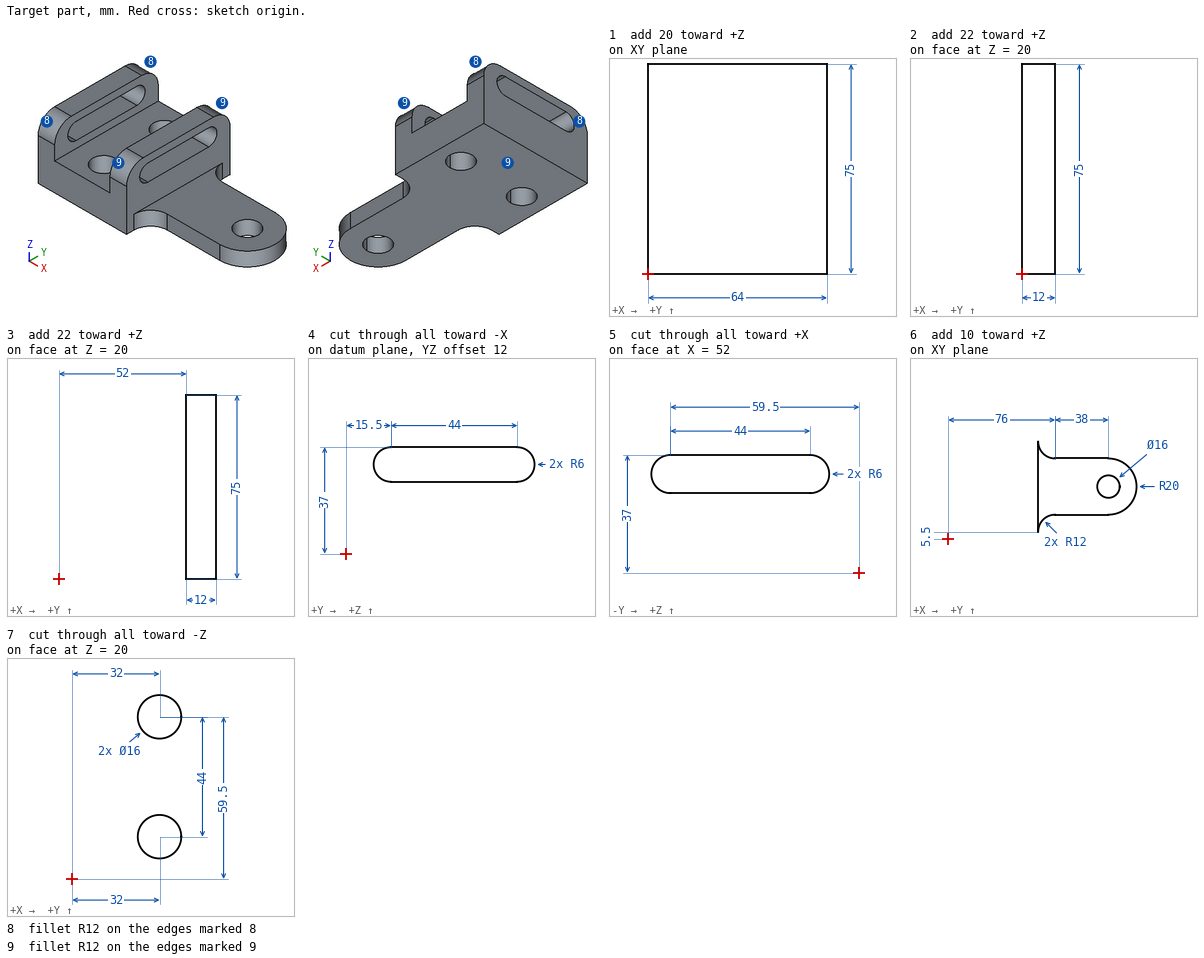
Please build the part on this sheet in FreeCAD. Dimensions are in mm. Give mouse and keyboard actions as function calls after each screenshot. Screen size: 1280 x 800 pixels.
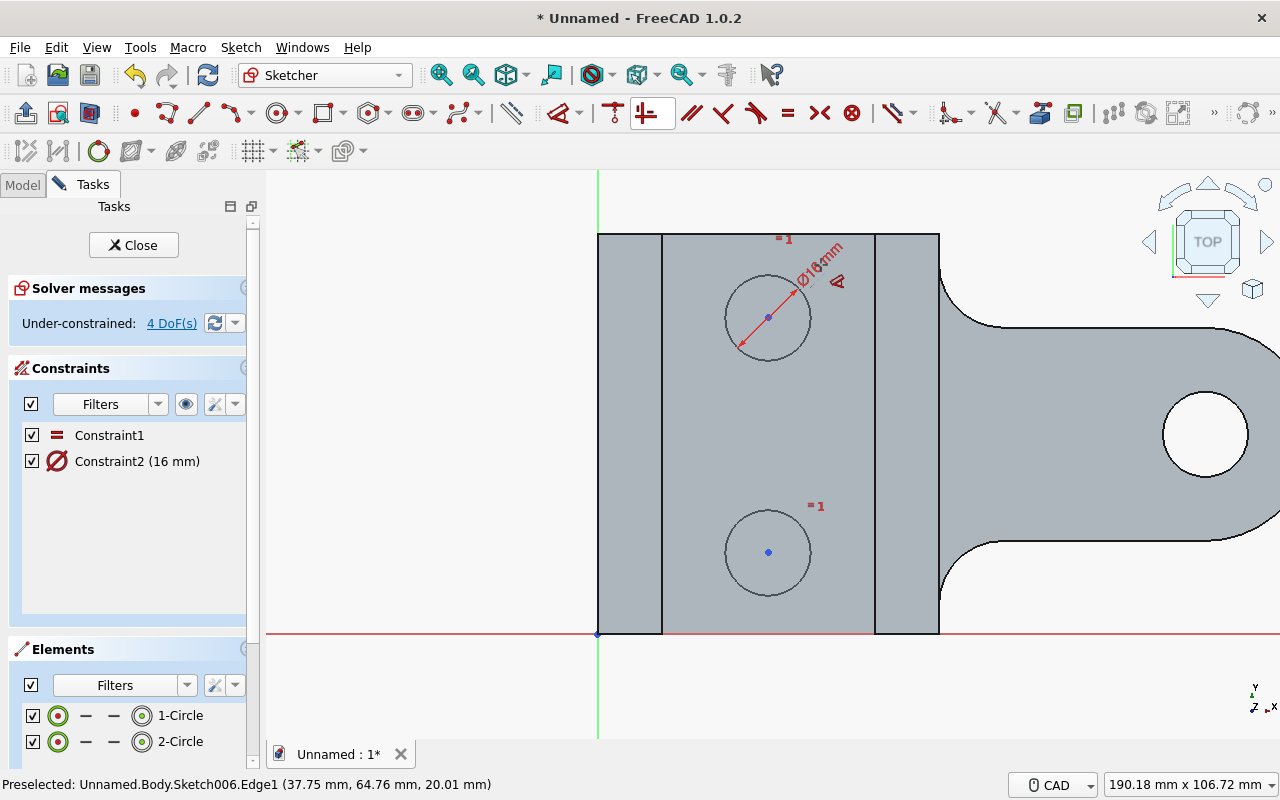
click(768, 318)
click(683, 668)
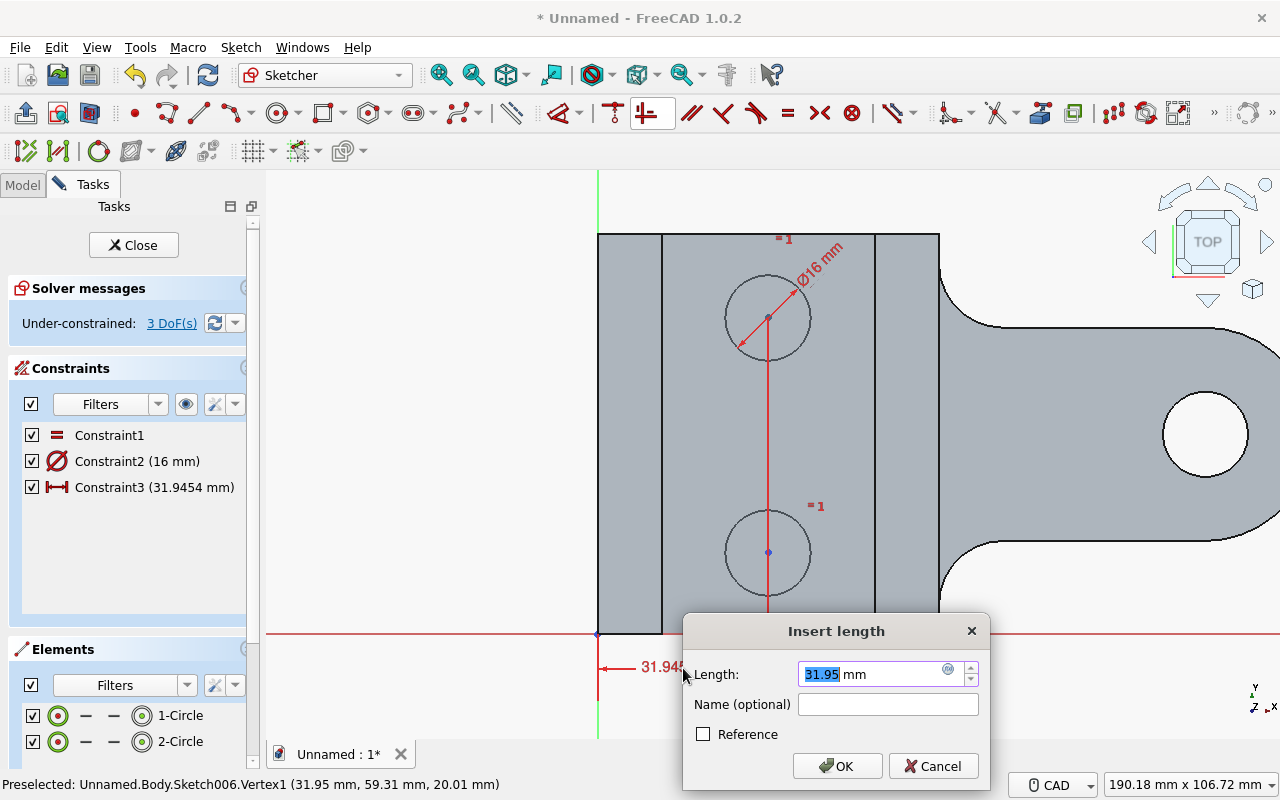
text(32)
key(Return)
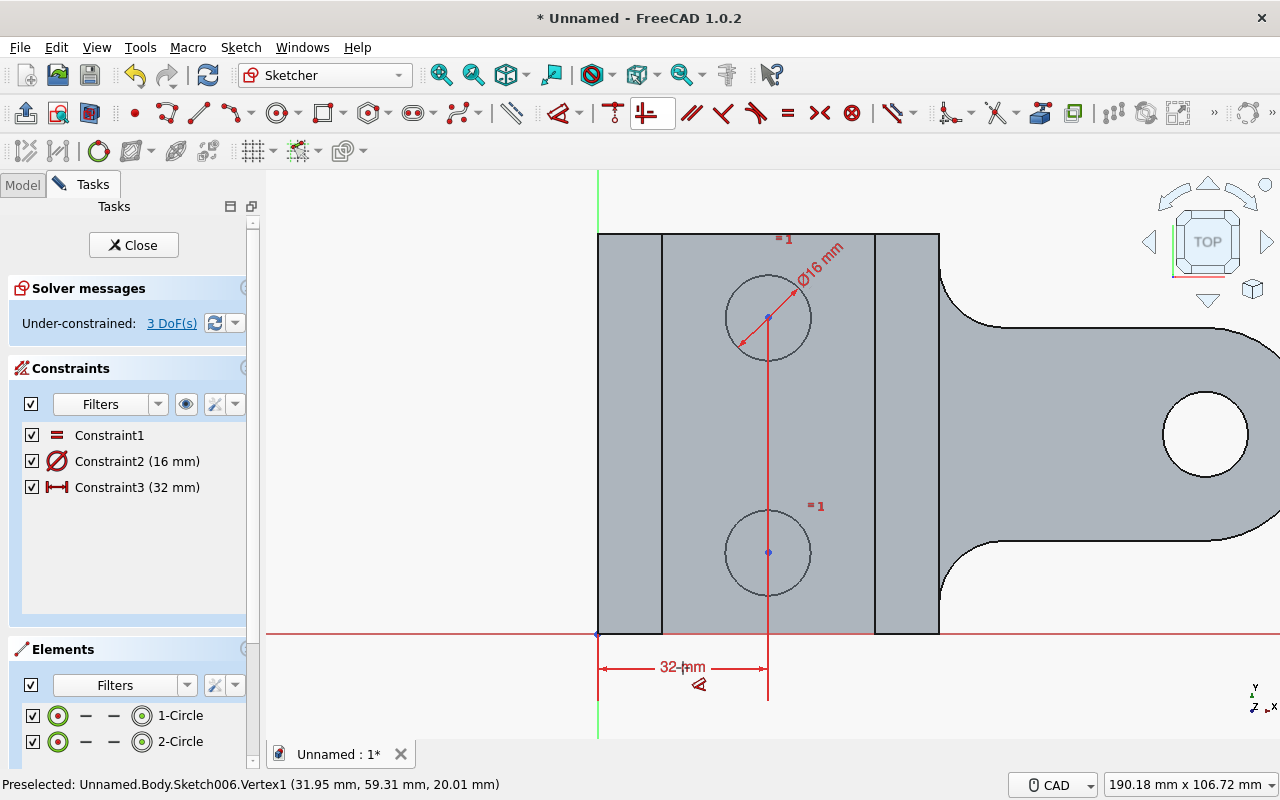
click(768, 553)
click(683, 519)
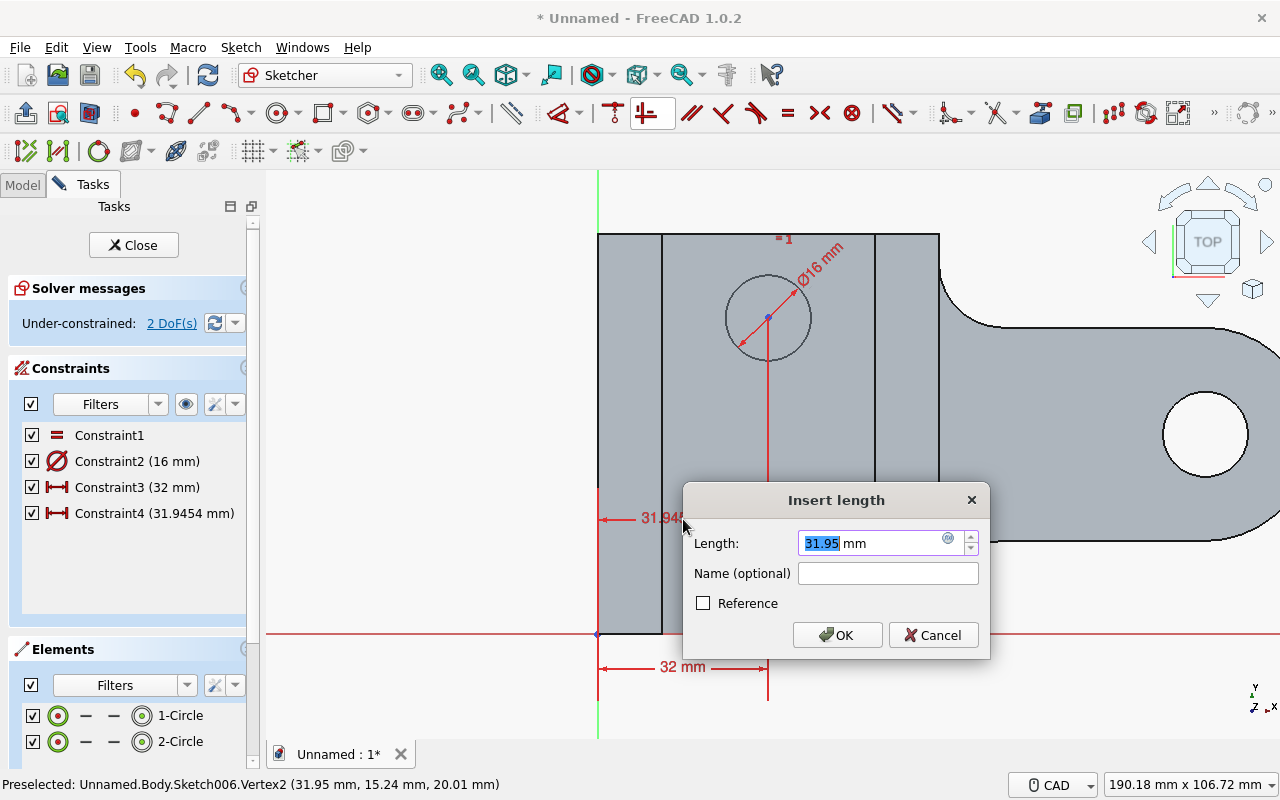
text(32)
key(Return)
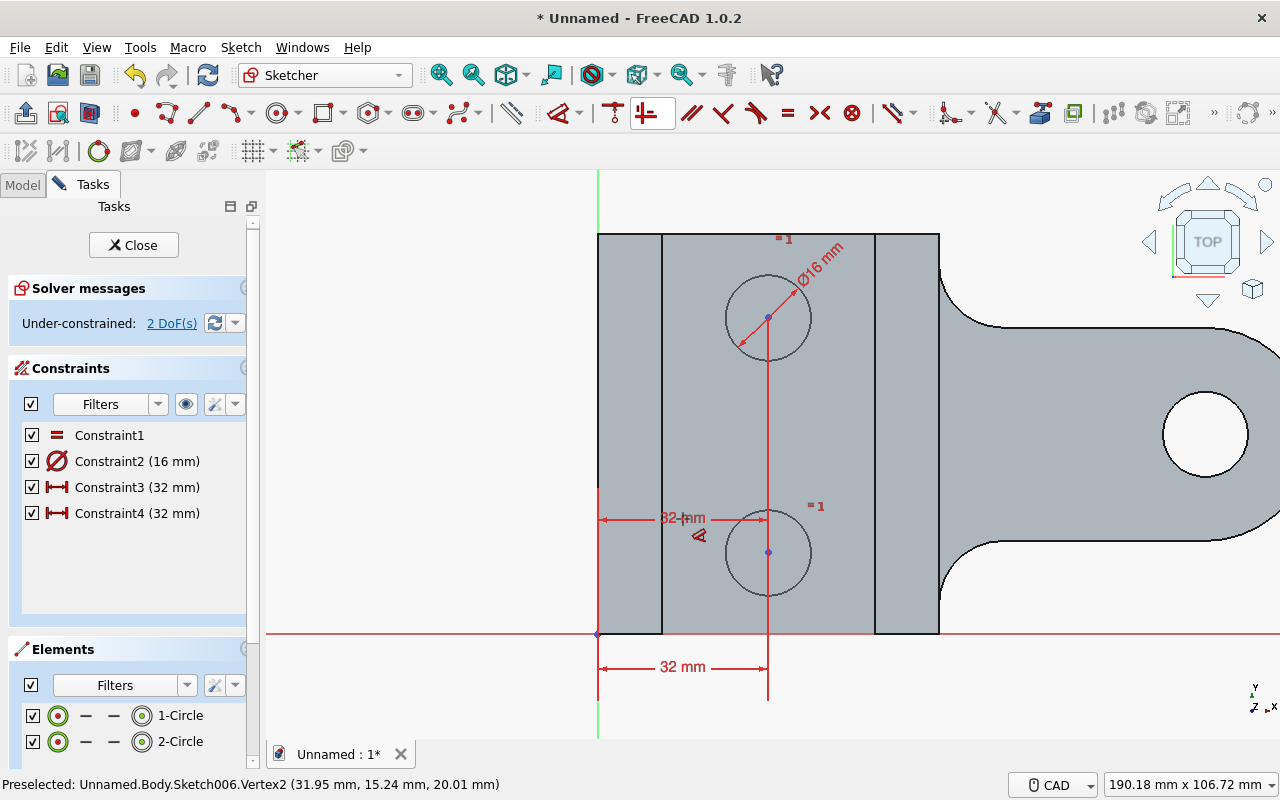
click(768, 318)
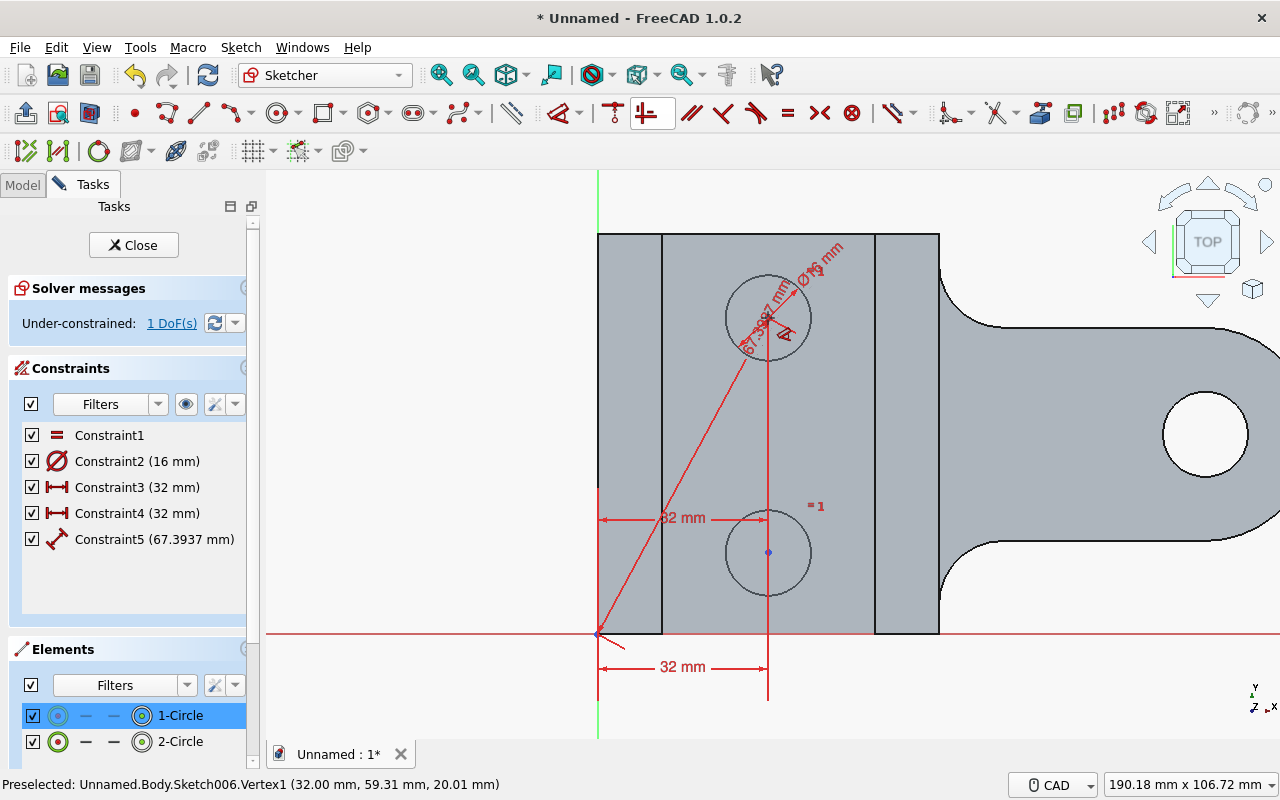
click(768, 553)
click(802, 435)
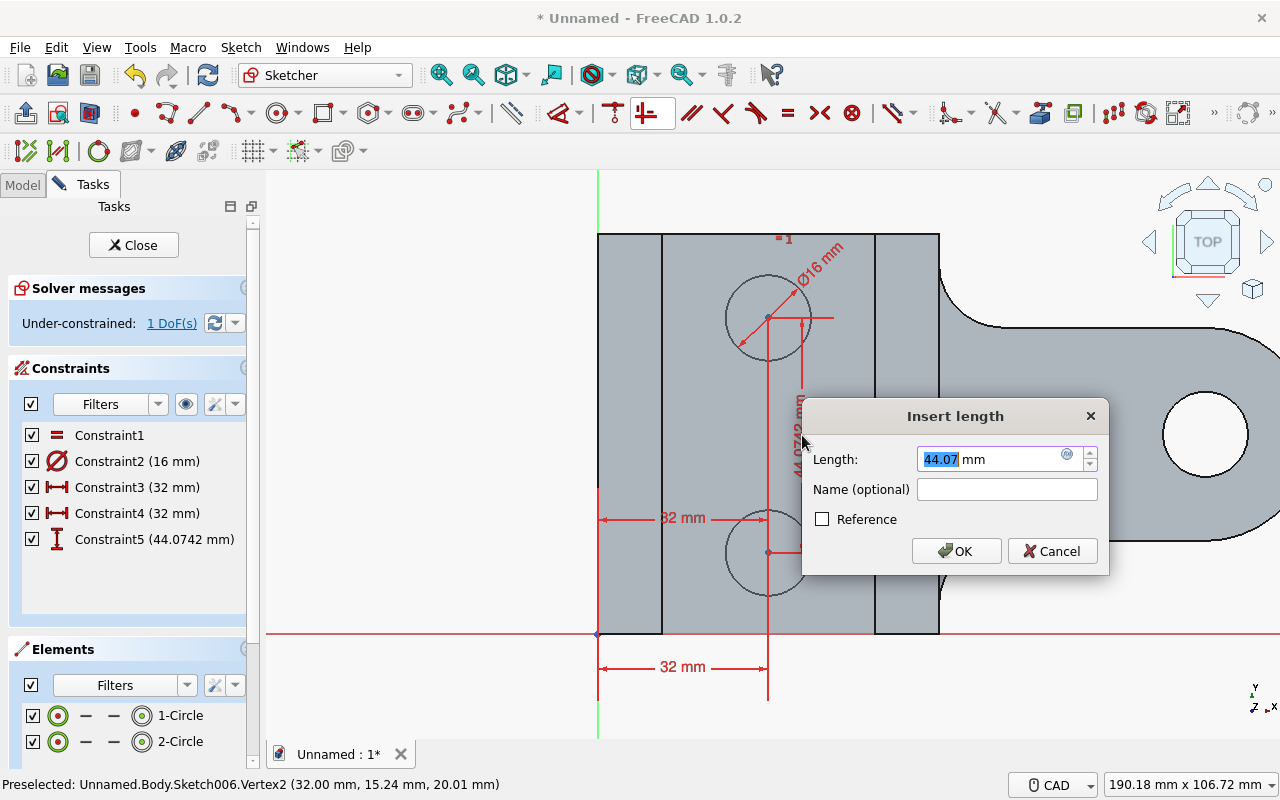
text(44)
key(Return)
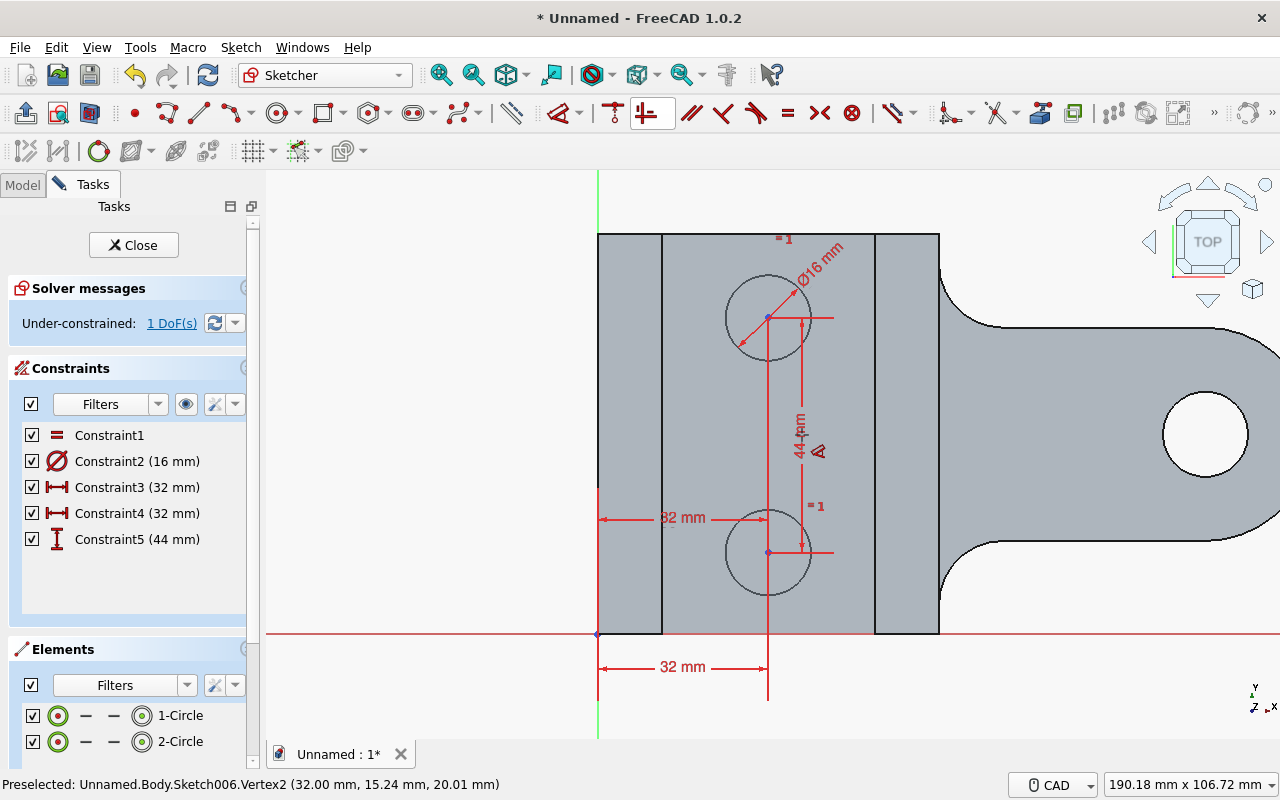
click(768, 318)
click(564, 476)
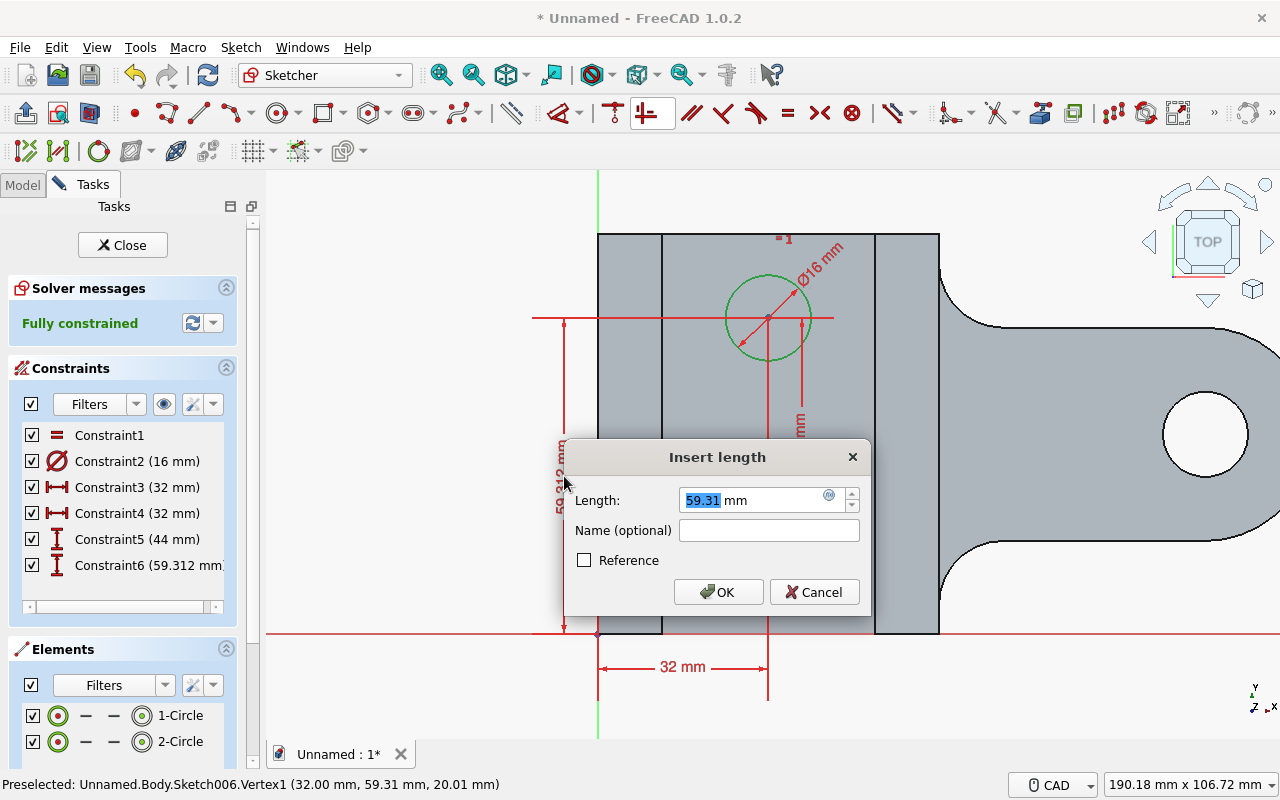
text(59.5)
key(Return)
key(Escape)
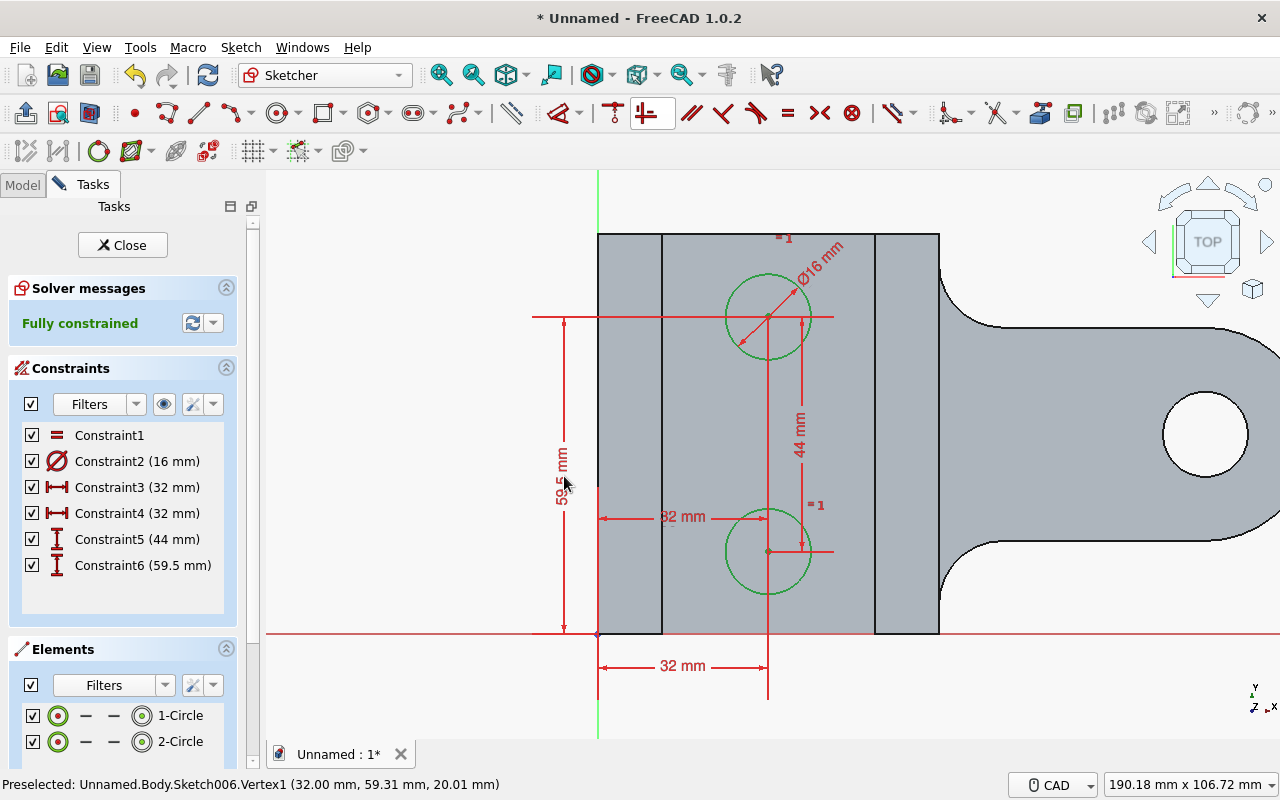
click(123, 245)